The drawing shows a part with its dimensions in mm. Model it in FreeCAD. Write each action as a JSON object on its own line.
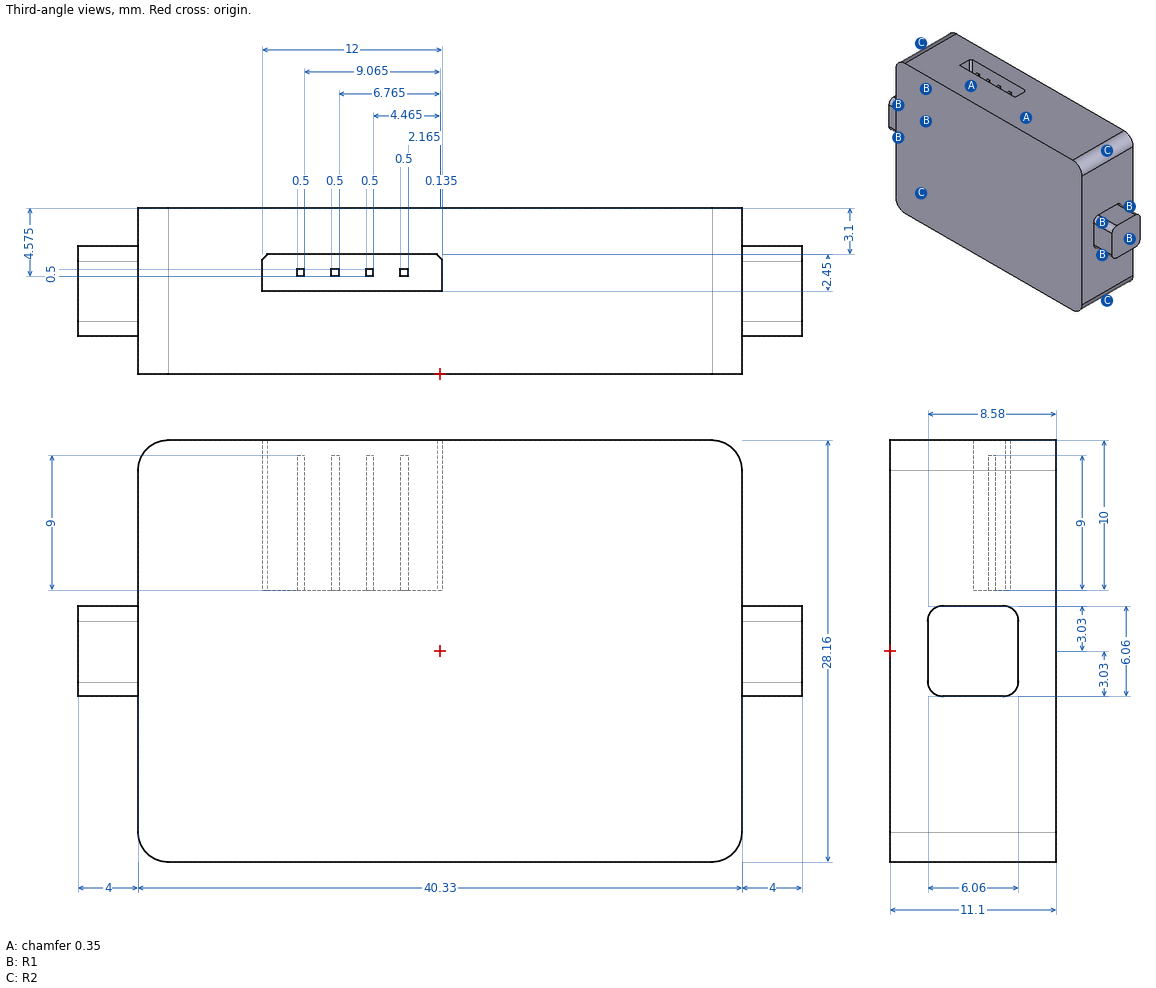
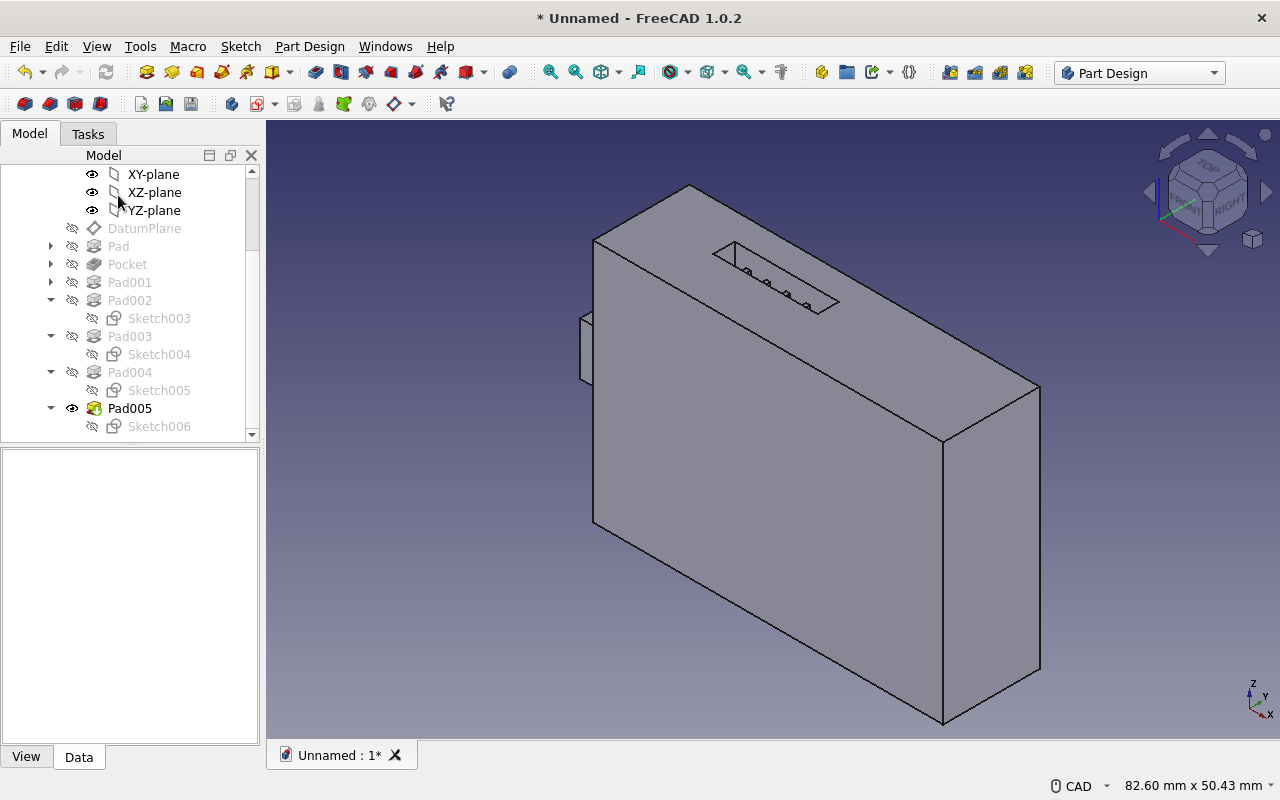
{"action": "left_click", "coordinate": [991, 555]}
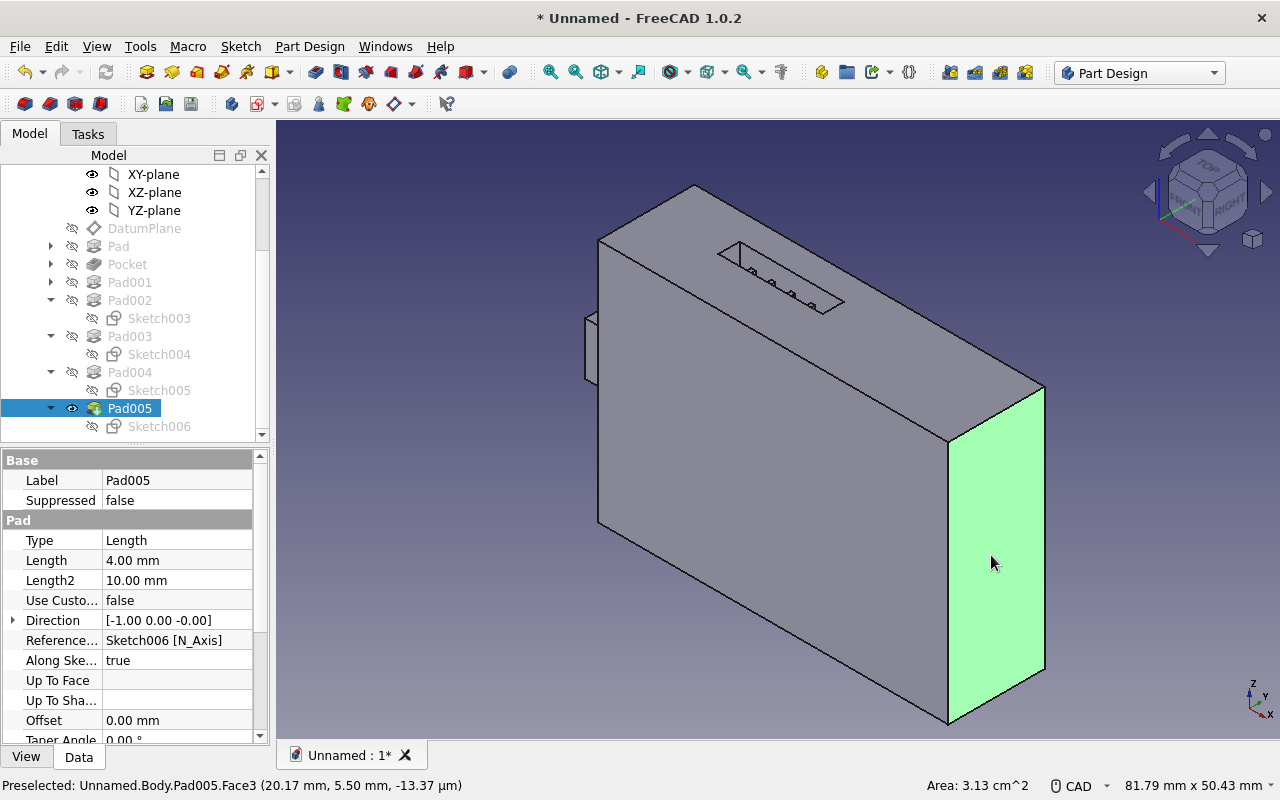
{"action": "left_click", "coordinate": [256, 104]}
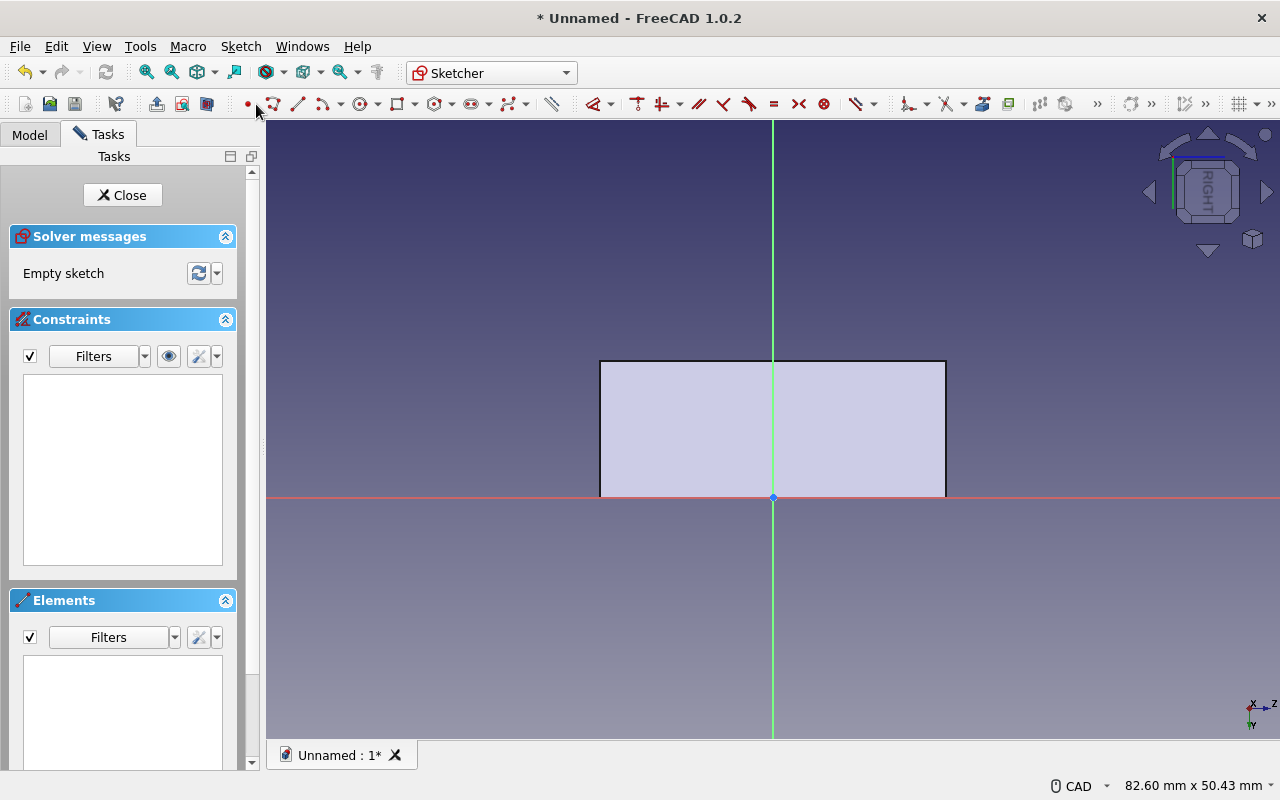
{"action": "scroll", "coordinate": [795, 450], "scroll_direction": "up", "scroll_amount": 7}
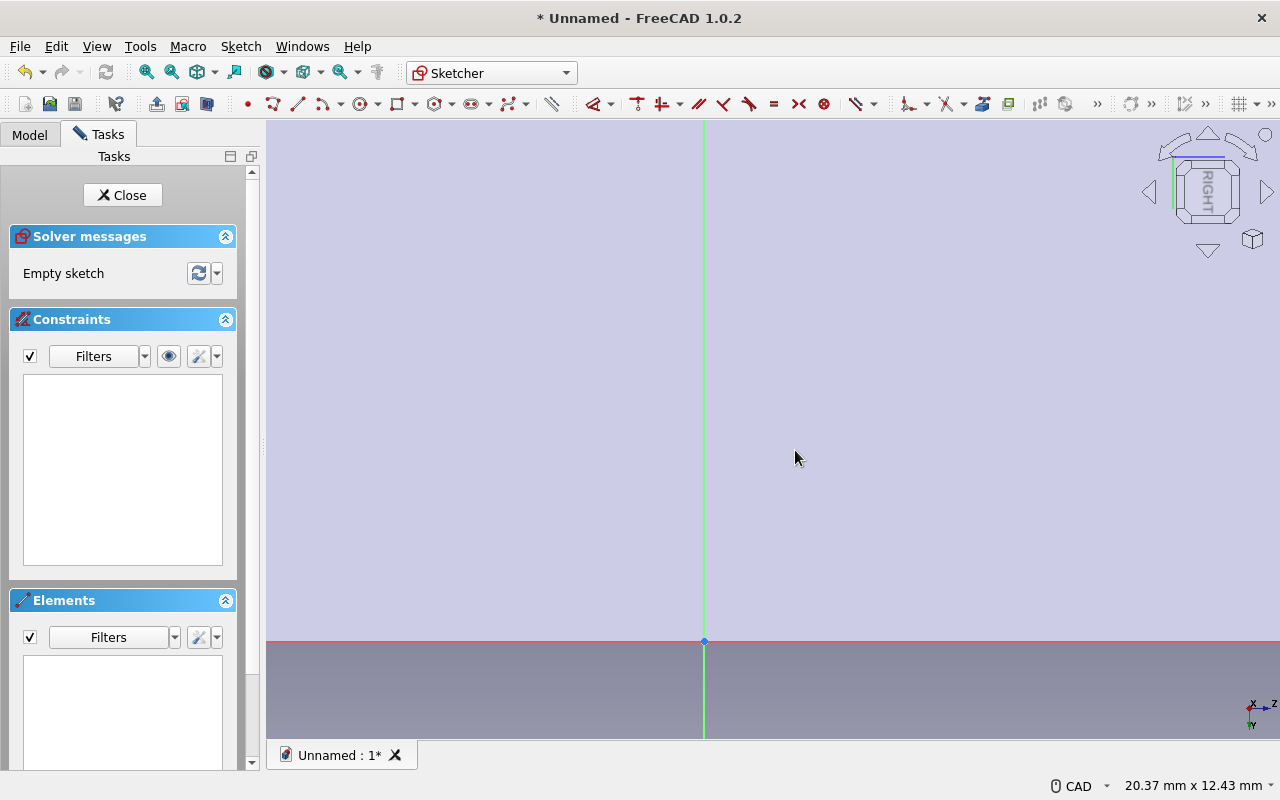
{"action": "key", "text": "g r"}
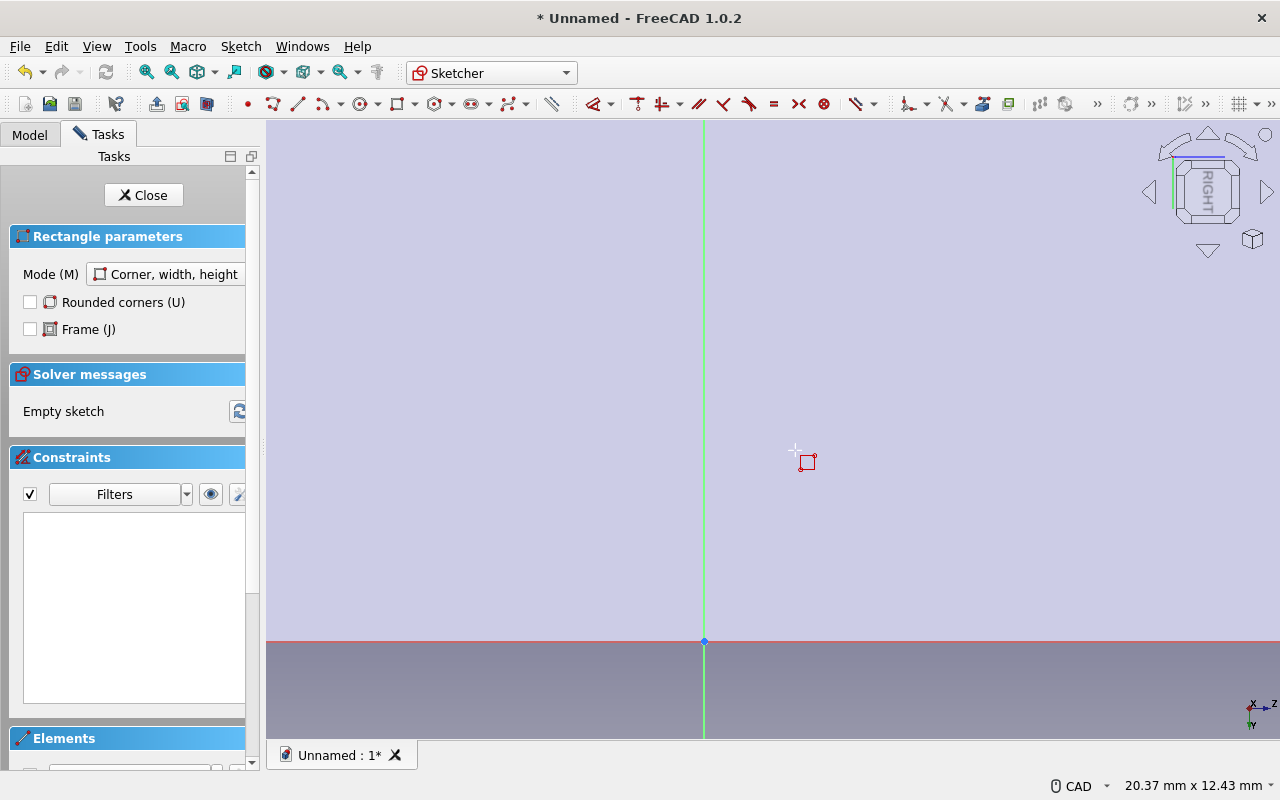
{"action": "left_click", "coordinate": [553, 214]}
{"action": "mouse_move", "coordinate": [855, 516]}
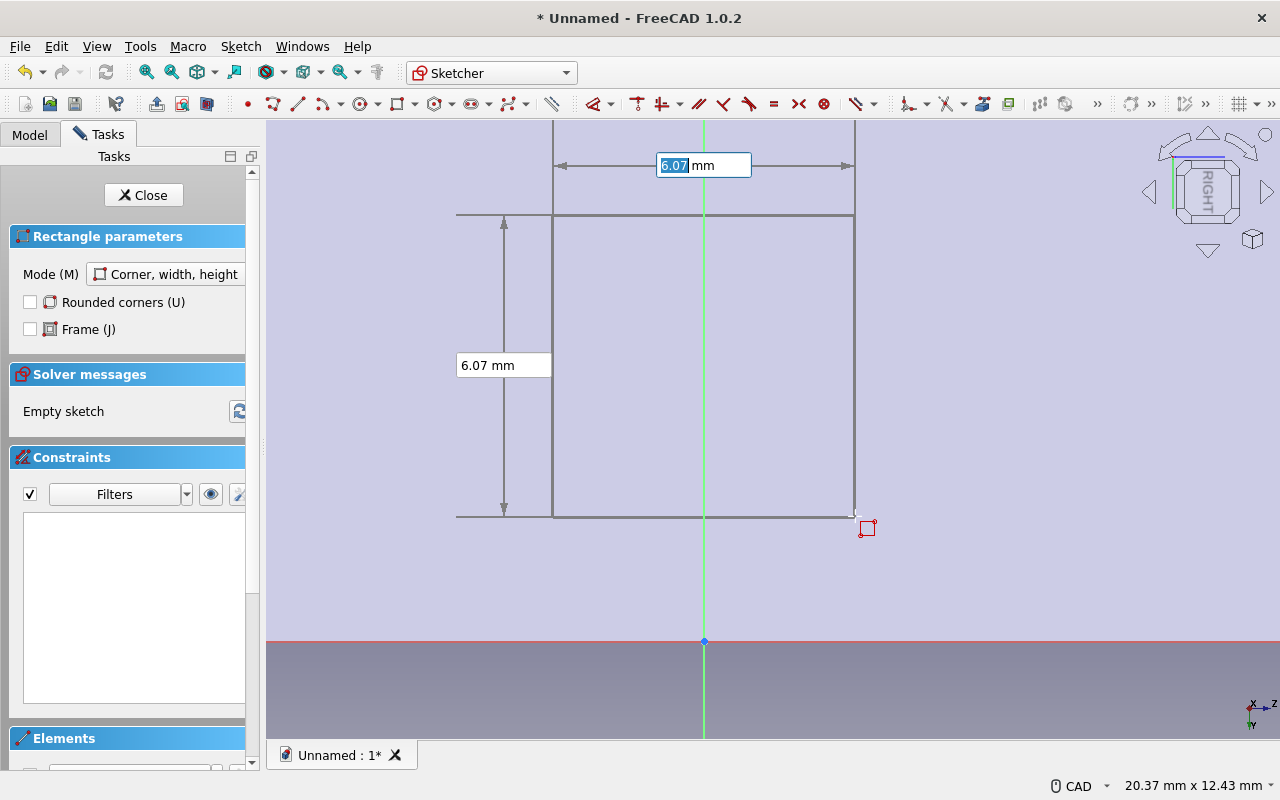
{"action": "type", "text": "6.06"}
{"action": "key", "text": "Tab"}
{"action": "type", "text": "6.06"}
{"action": "key", "text": "Return"}
{"action": "key", "text": "Escape"}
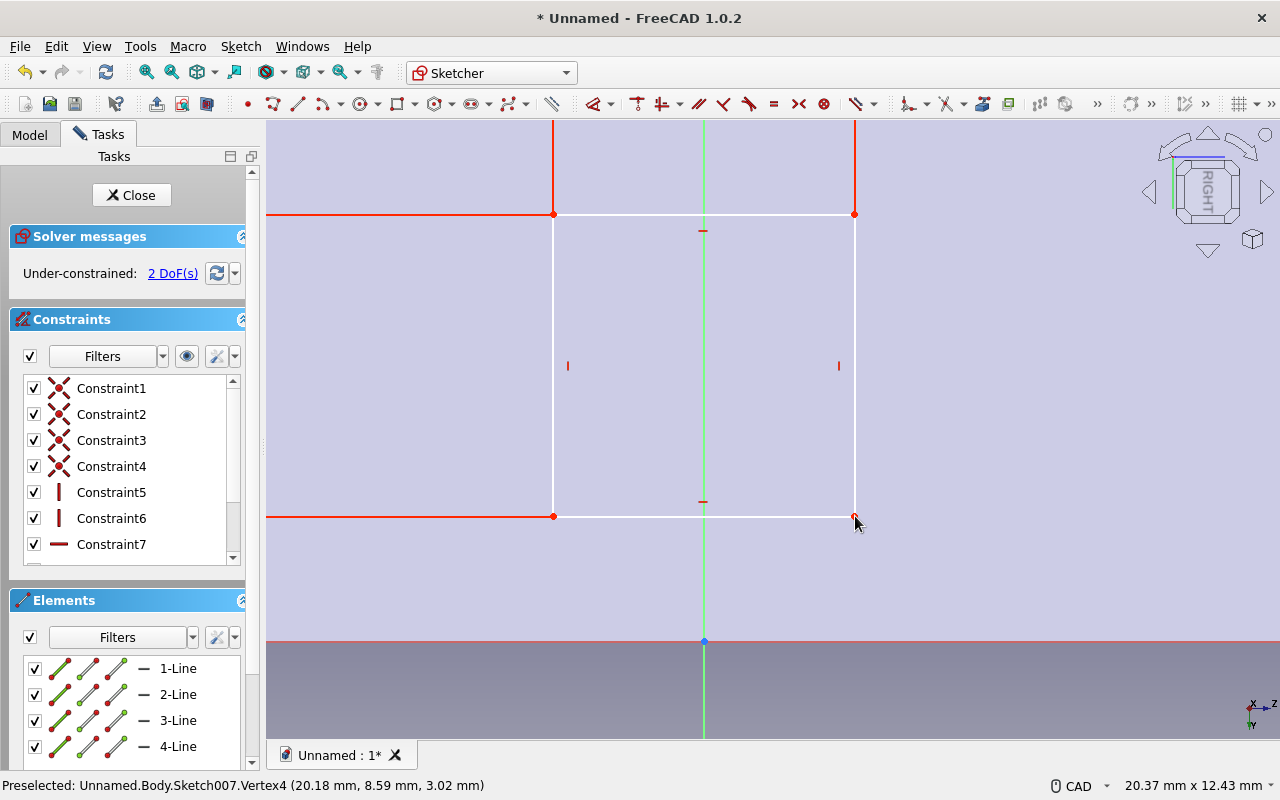
{"action": "key", "text": "d"}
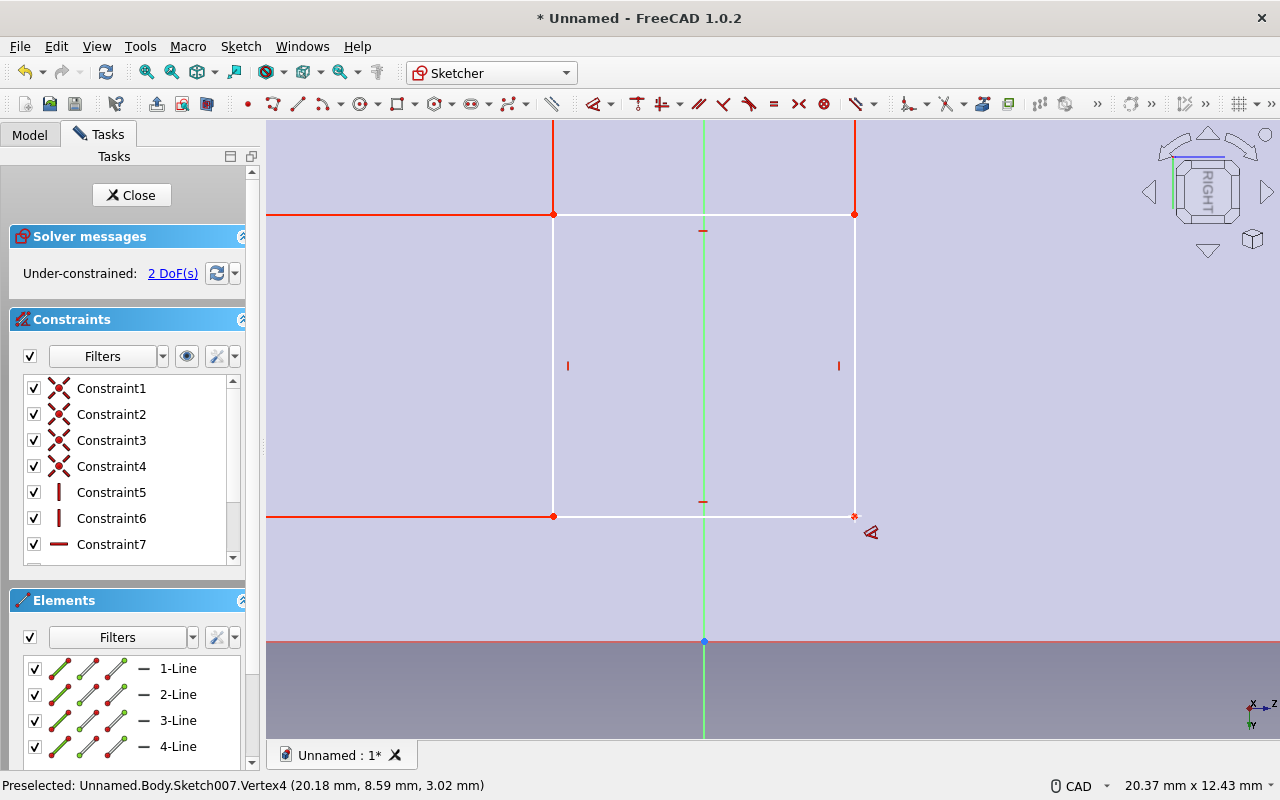
{"action": "left_click", "coordinate": [553, 215]}
{"action": "left_click", "coordinate": [629, 676]}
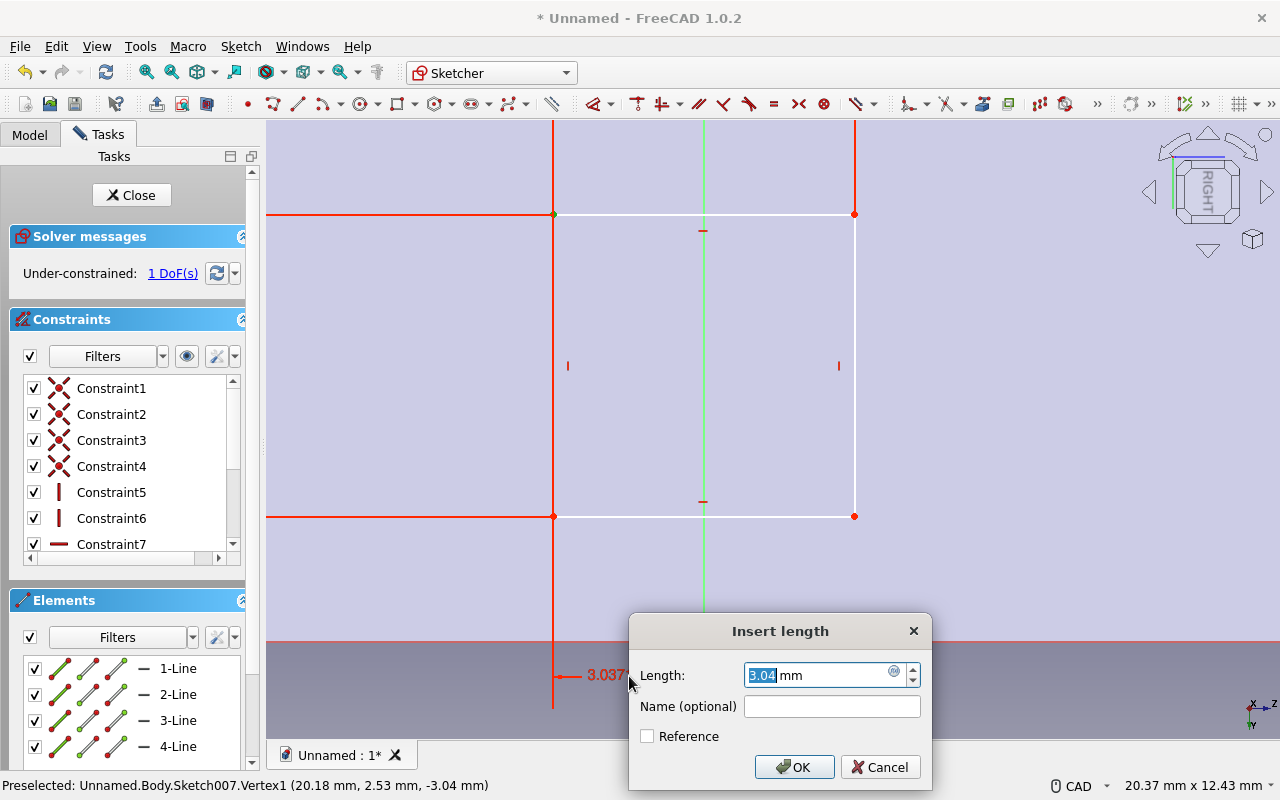
{"action": "type", "text": "3.03"}
{"action": "key", "text": "Return"}